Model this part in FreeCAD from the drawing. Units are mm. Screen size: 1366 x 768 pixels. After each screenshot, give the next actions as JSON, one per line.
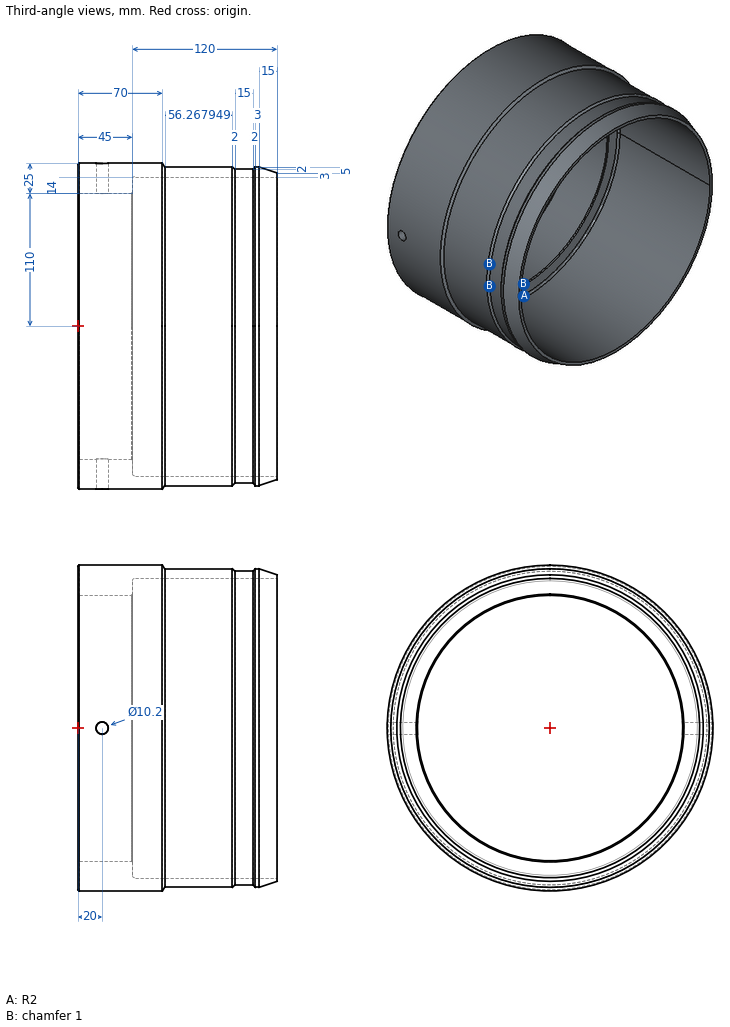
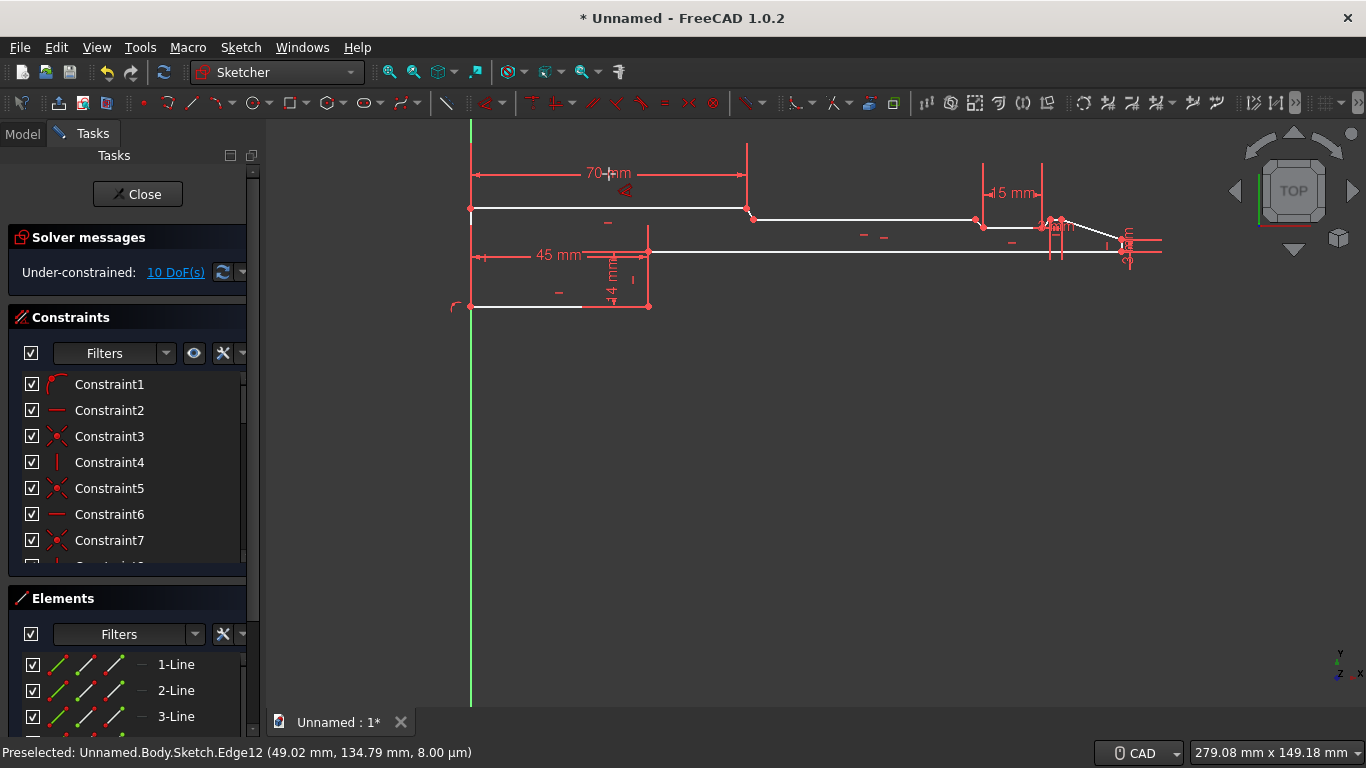
{"action": "left_click", "coordinate": [471, 238]}
{"action": "left_click", "coordinate": [437, 258]}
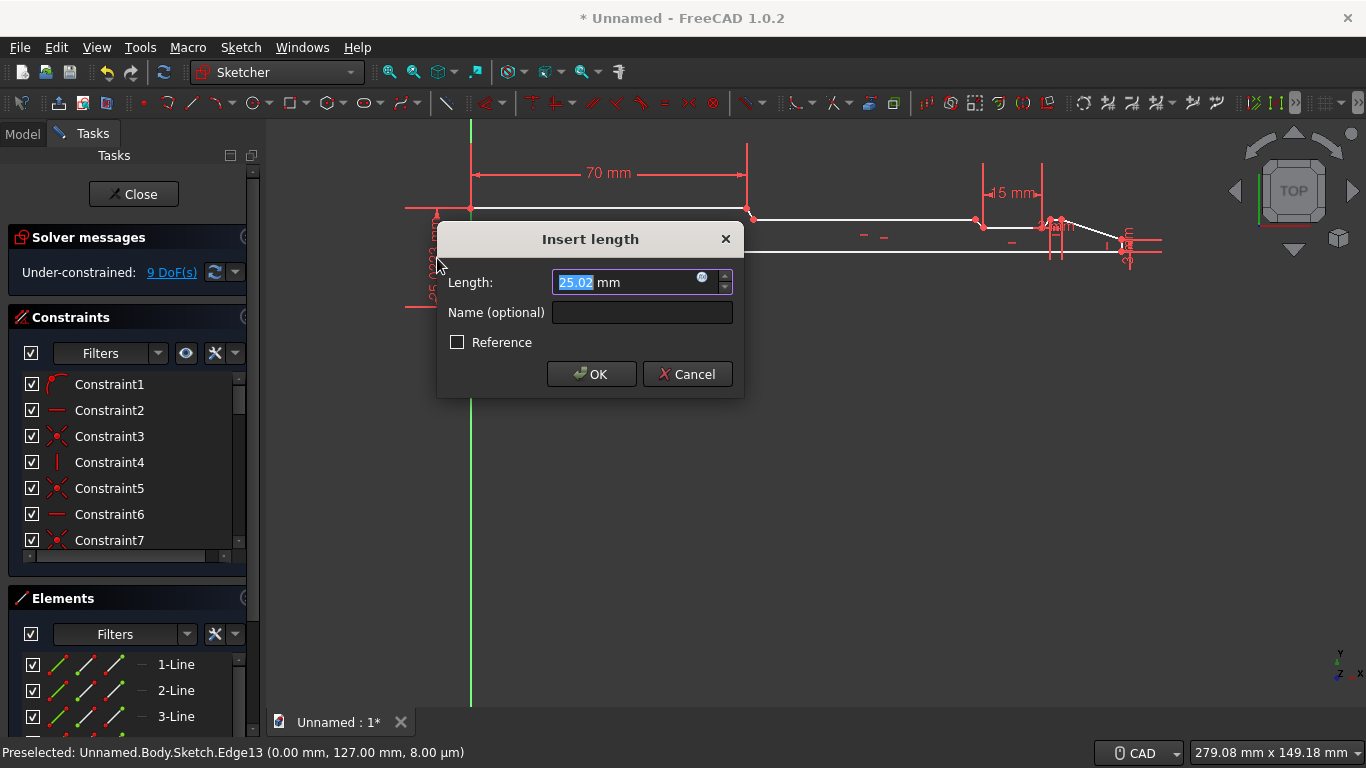
{"action": "type", "text": "25"}
{"action": "key", "text": "Return"}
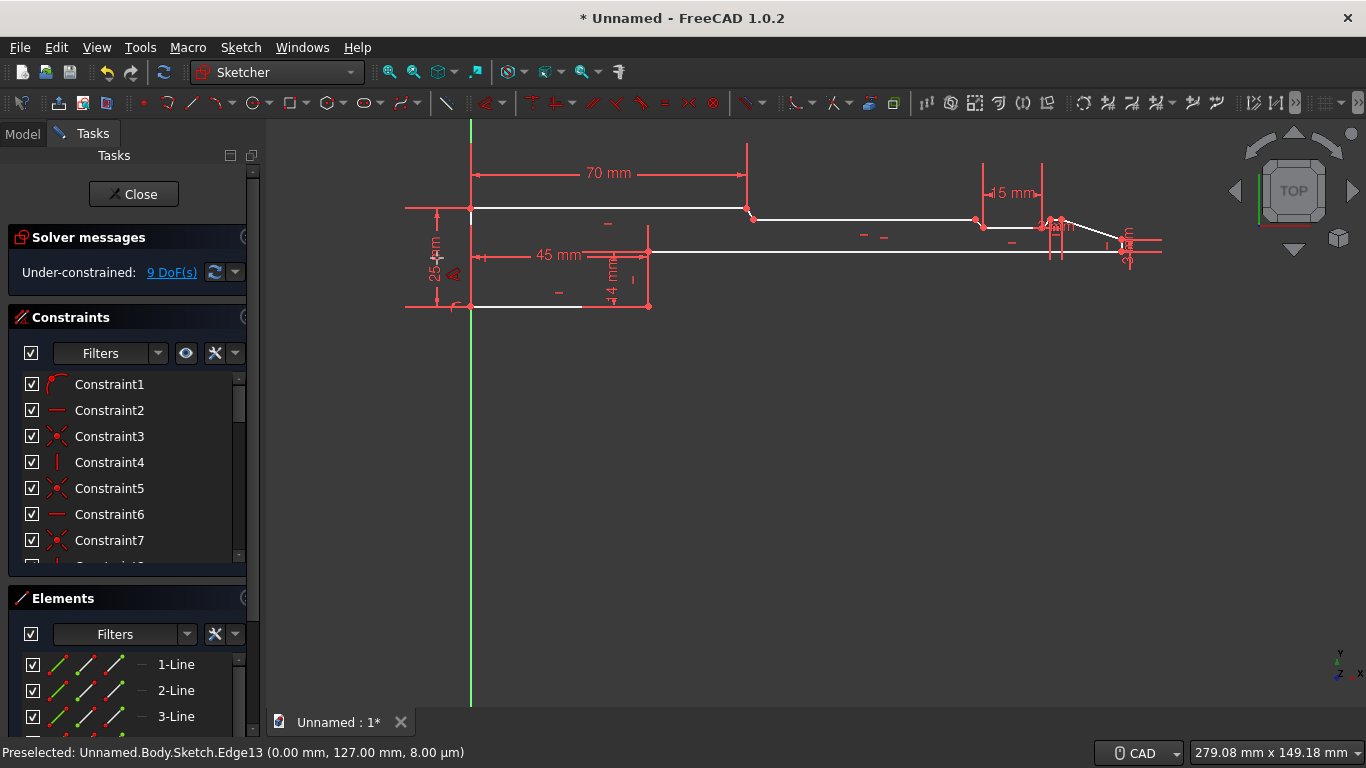
{"action": "scroll", "coordinate": [1104, 234], "scroll_direction": "up", "scroll_amount": 4}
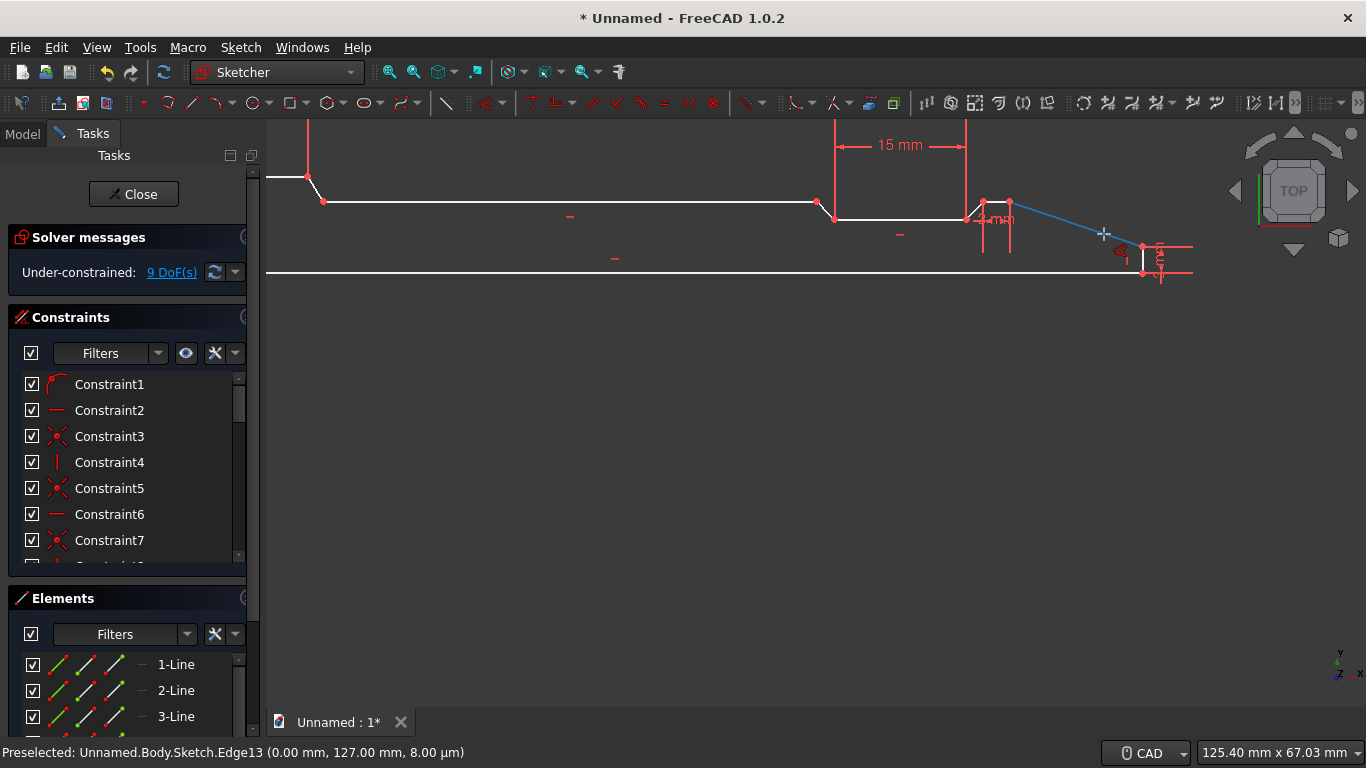
{"action": "left_click", "coordinate": [1103, 233]}
{"action": "left_click", "coordinate": [1177, 224]}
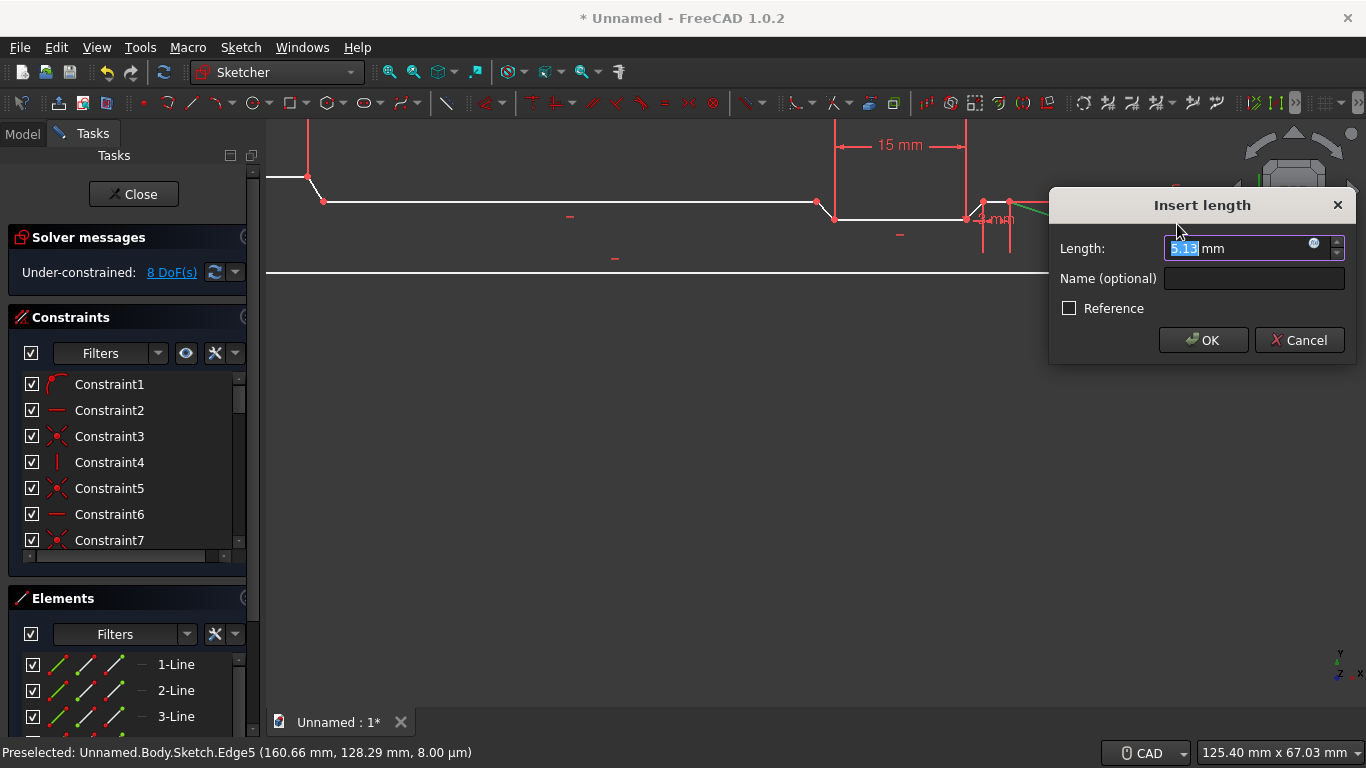
{"action": "type", "text": "5"}
{"action": "key", "text": "Return"}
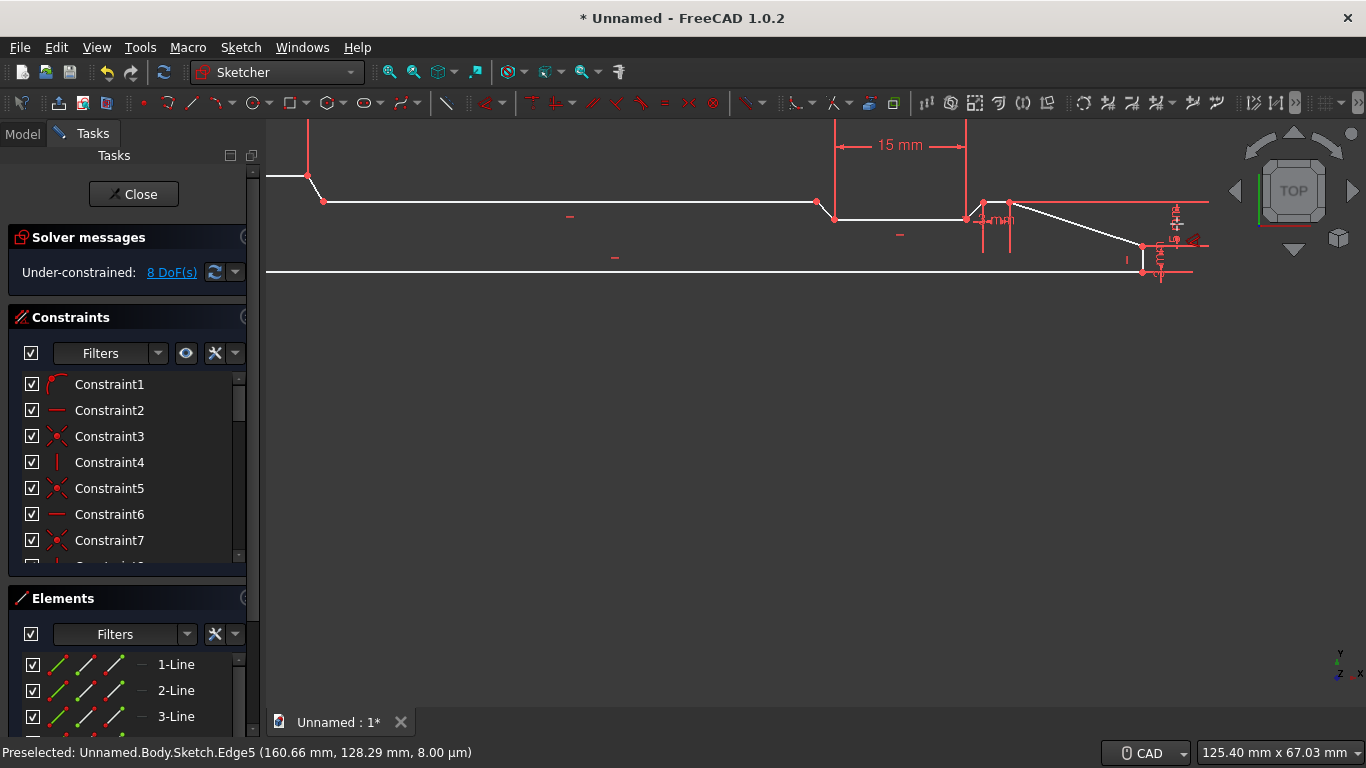
{"action": "scroll", "coordinate": [976, 209], "scroll_direction": "up", "scroll_amount": 5}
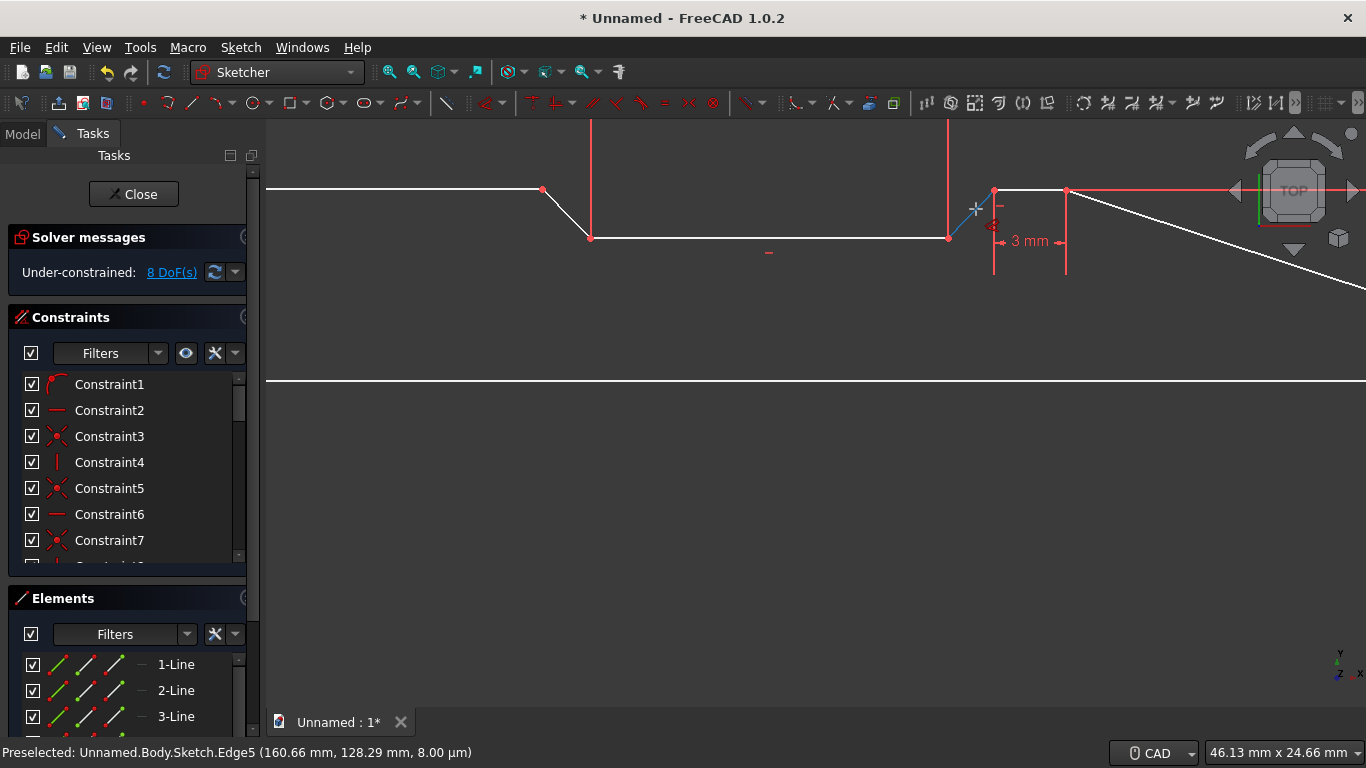
{"action": "left_click", "coordinate": [976, 209]}
{"action": "left_click", "coordinate": [971, 156]}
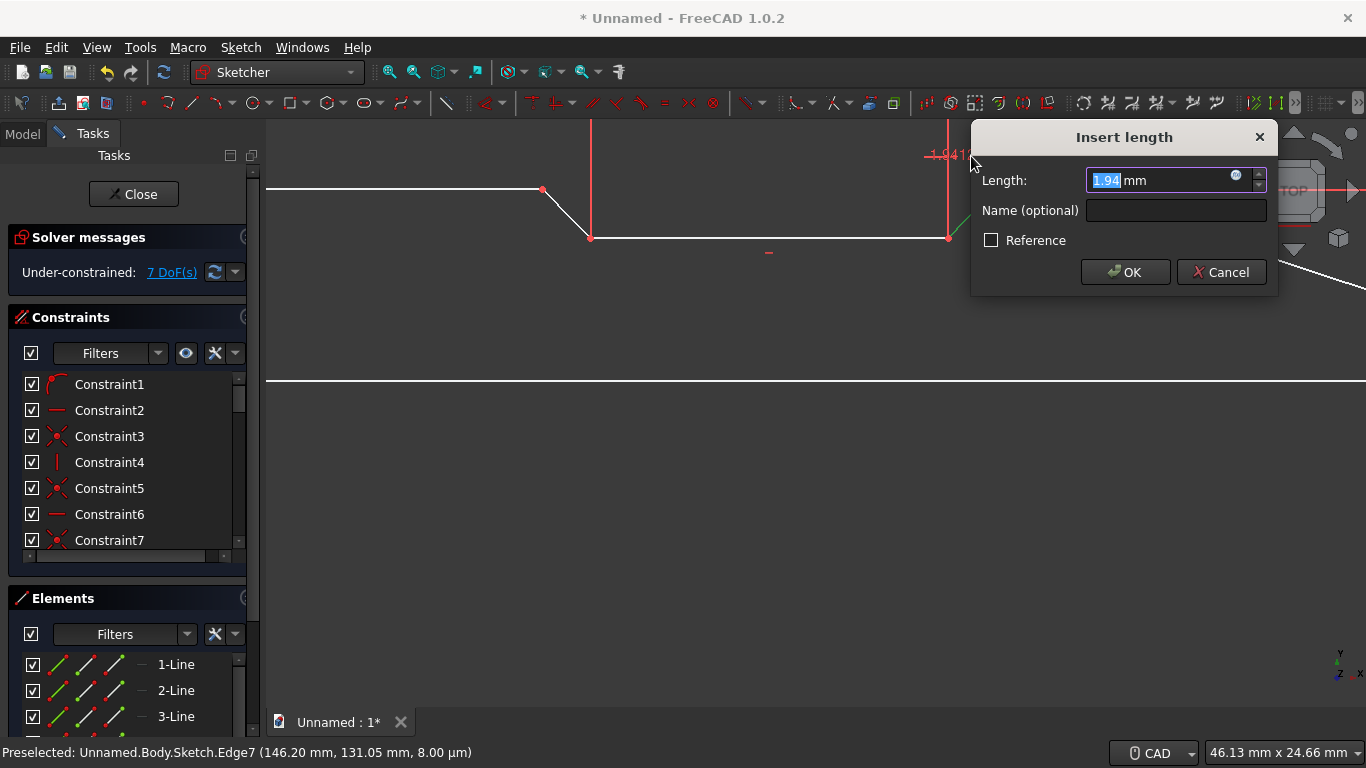
{"action": "type", "text": "2"}
{"action": "key", "text": "Return"}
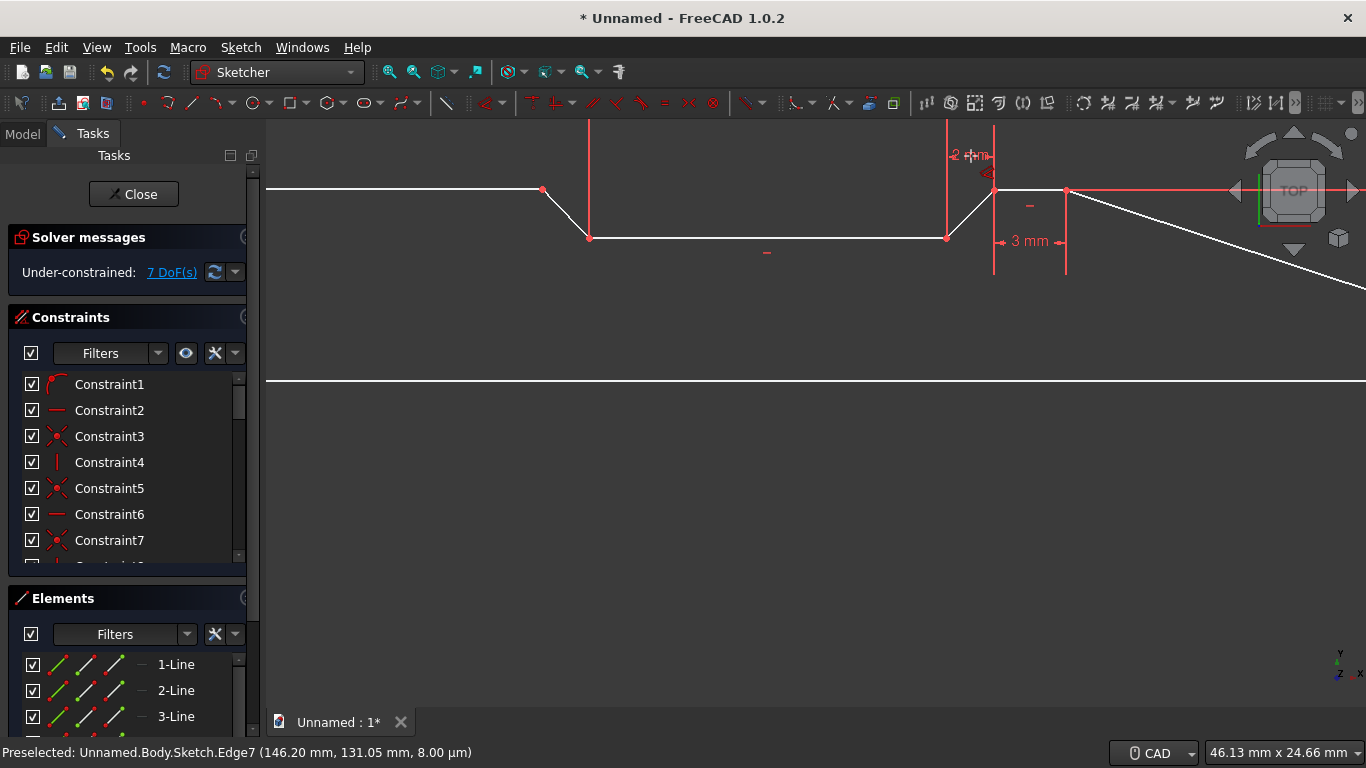
{"action": "left_click", "coordinate": [980, 205]}
{"action": "left_click", "coordinate": [1028, 214]}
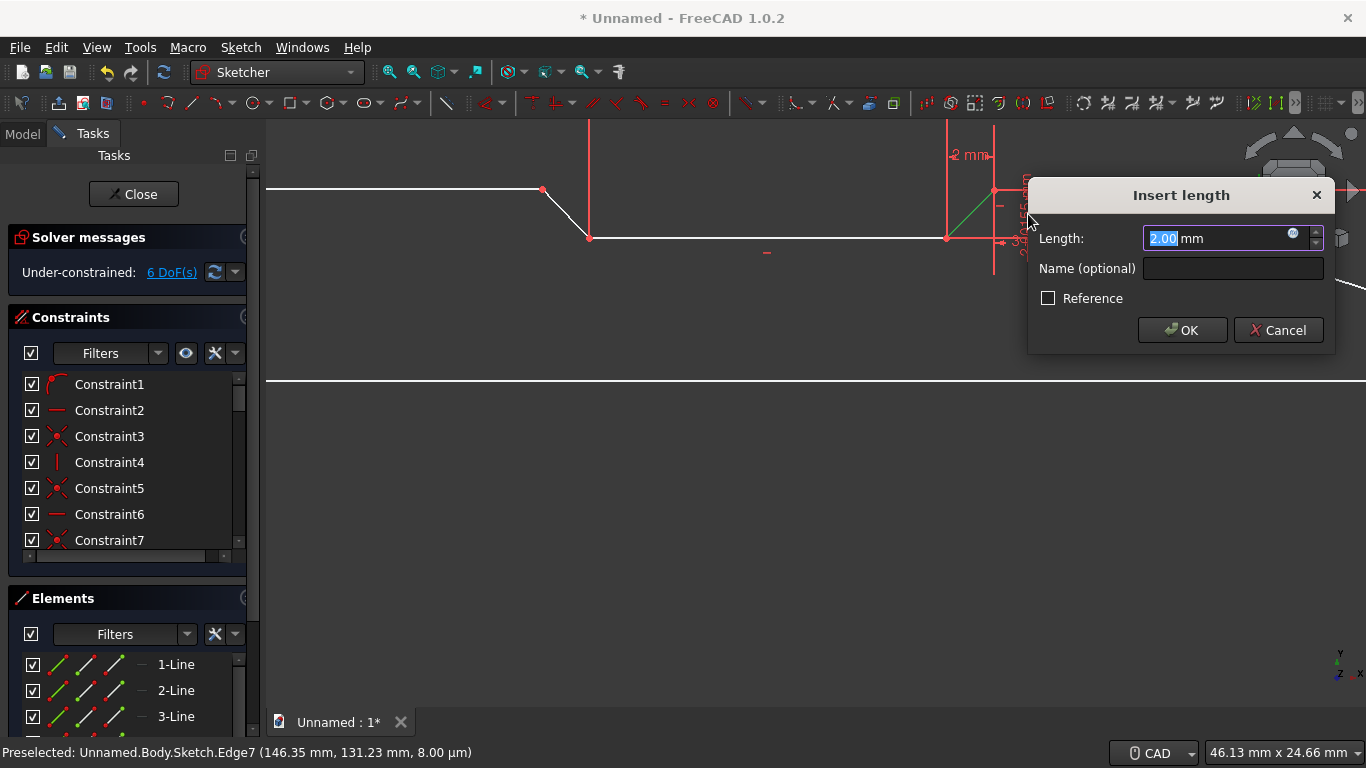
{"action": "type", "text": "2"}
{"action": "key", "text": "Return"}